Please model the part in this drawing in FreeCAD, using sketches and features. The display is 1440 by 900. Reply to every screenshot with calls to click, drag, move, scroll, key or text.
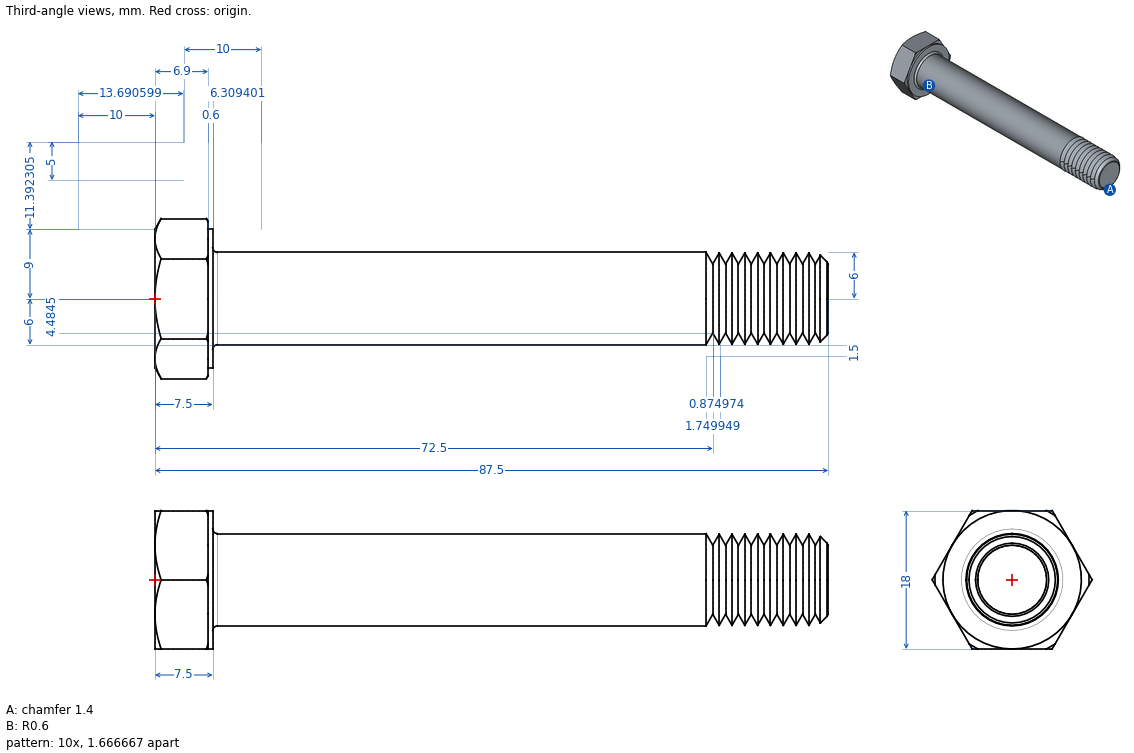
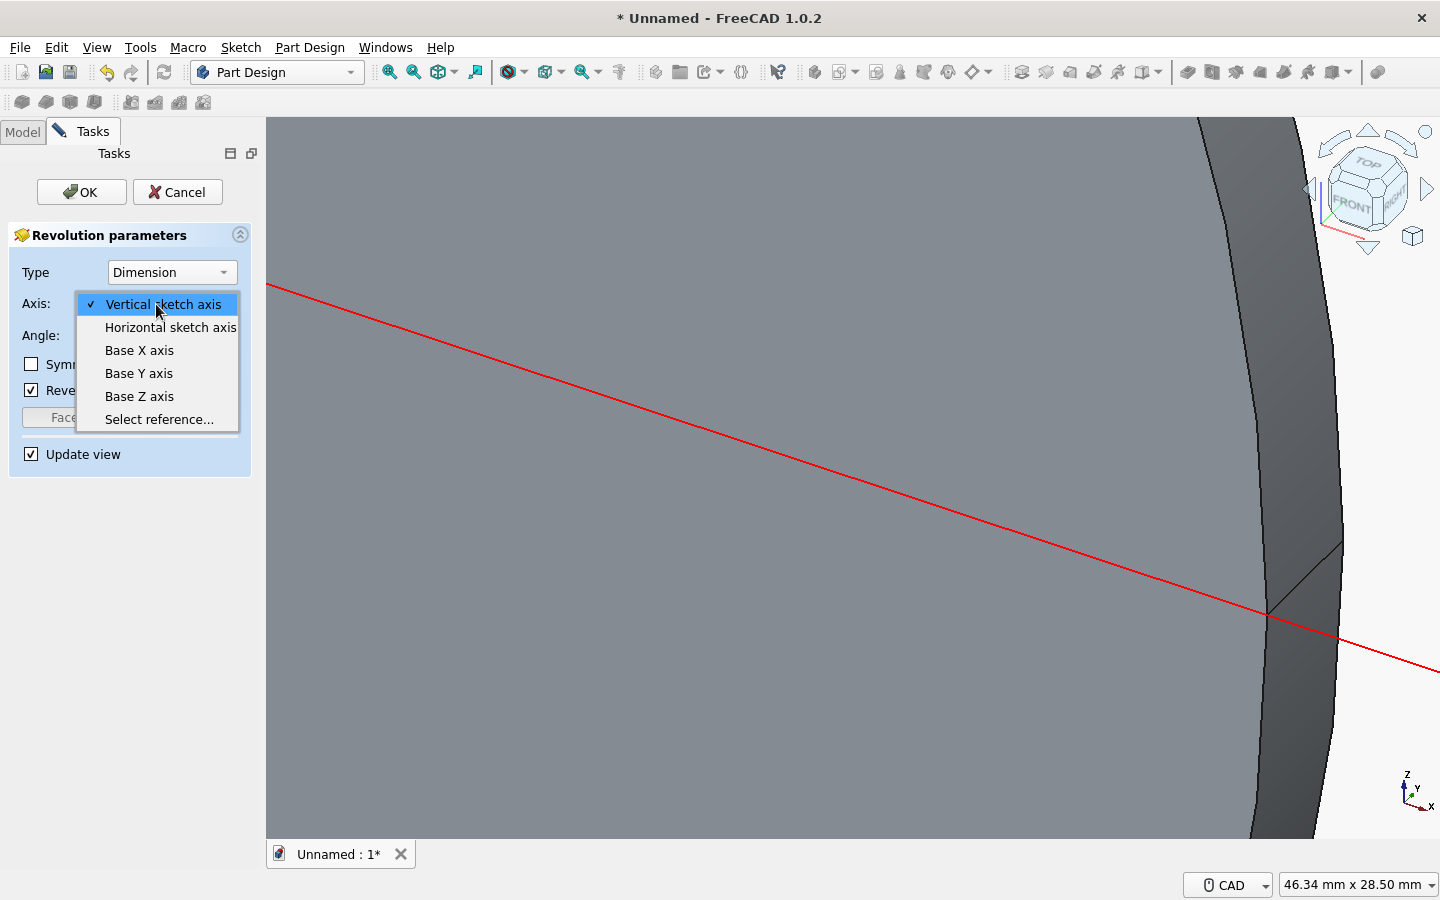
click(156, 328)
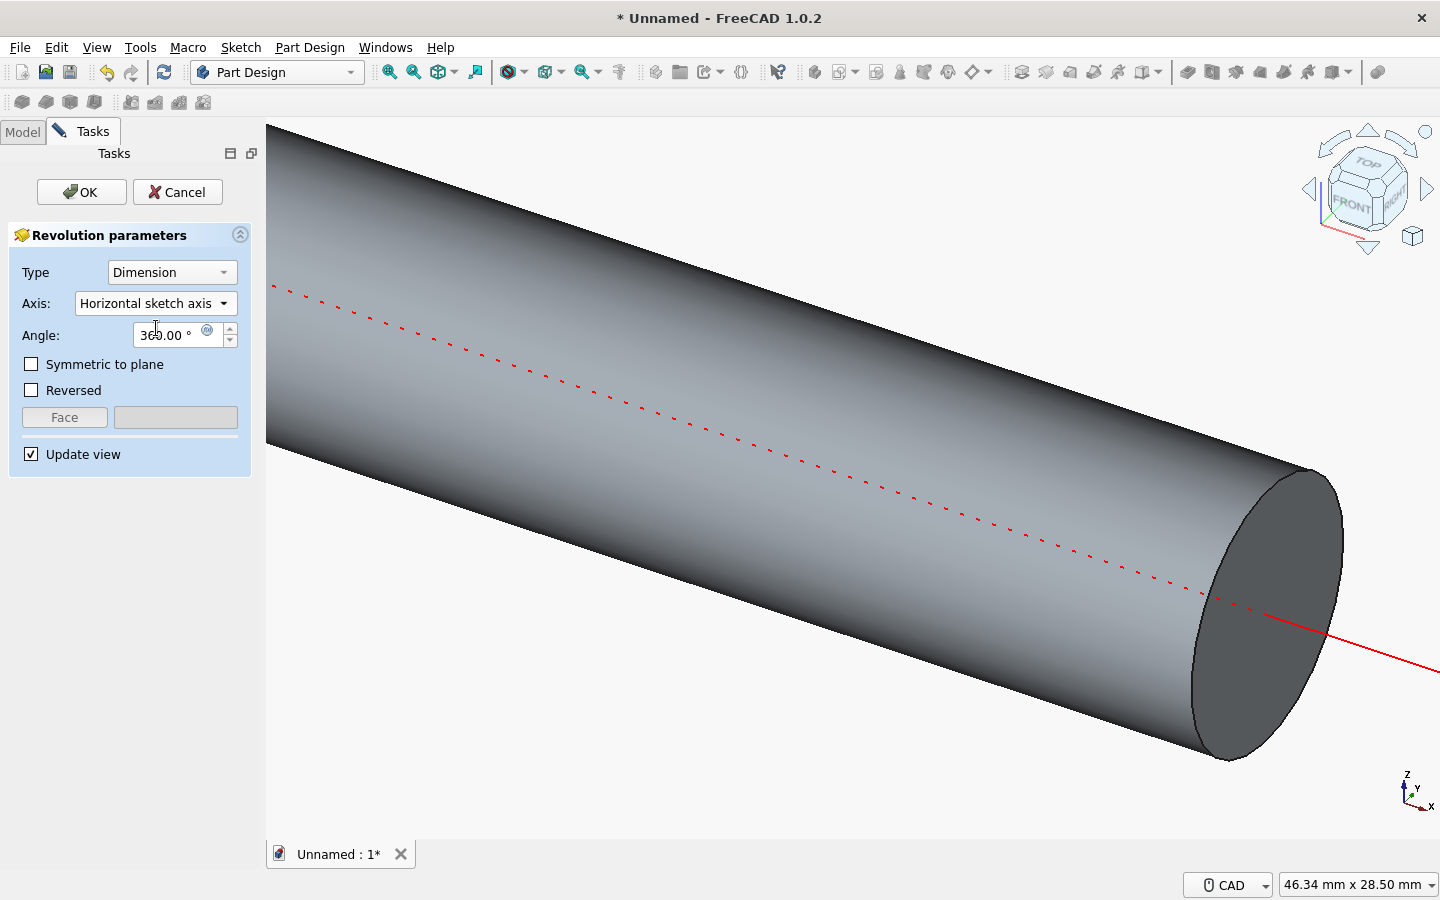
click(82, 192)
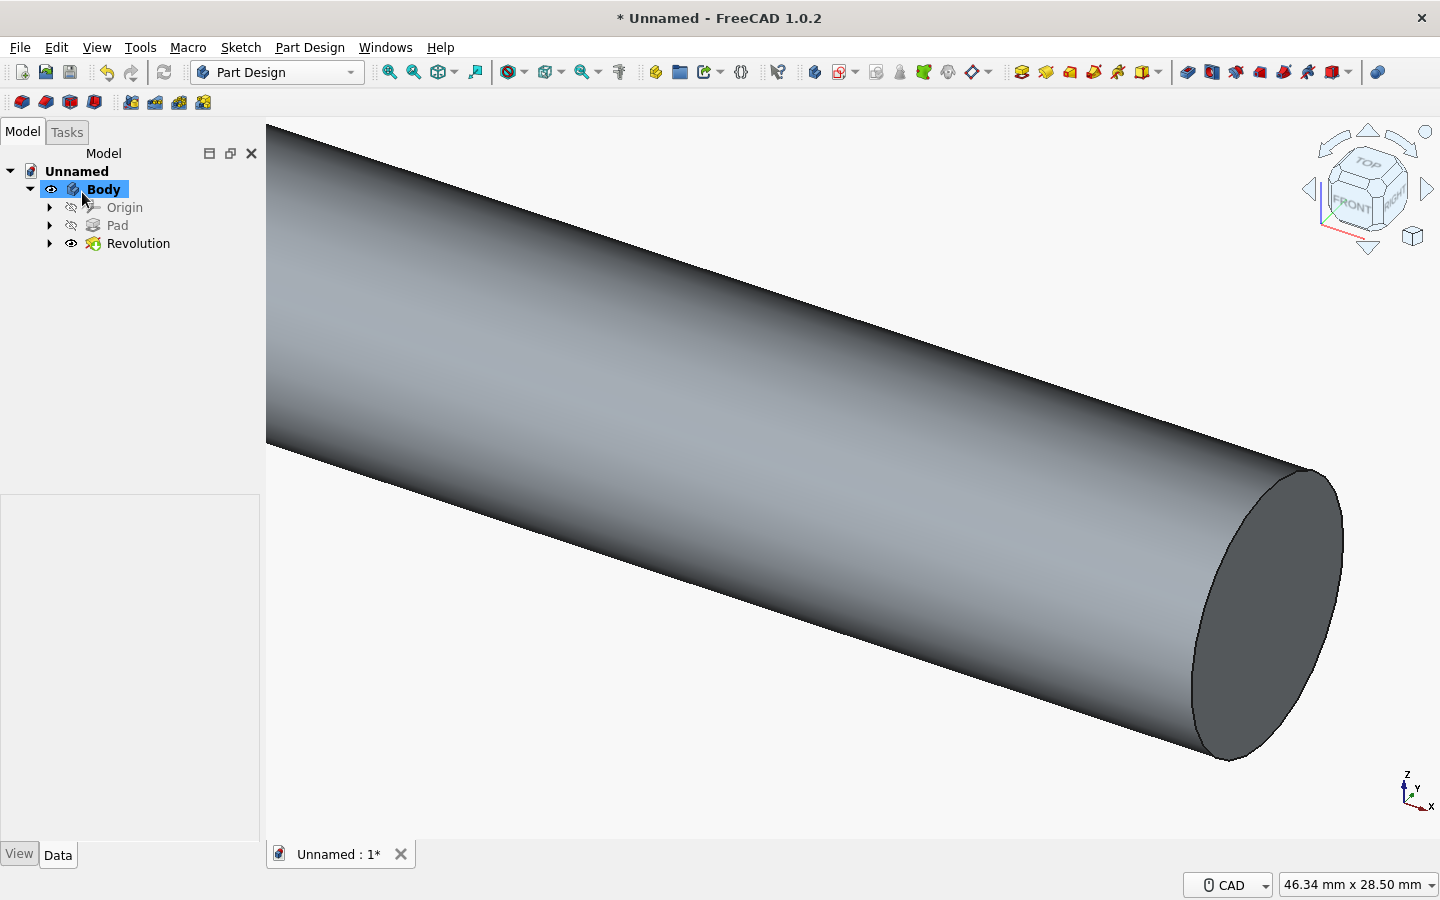
click(390, 72)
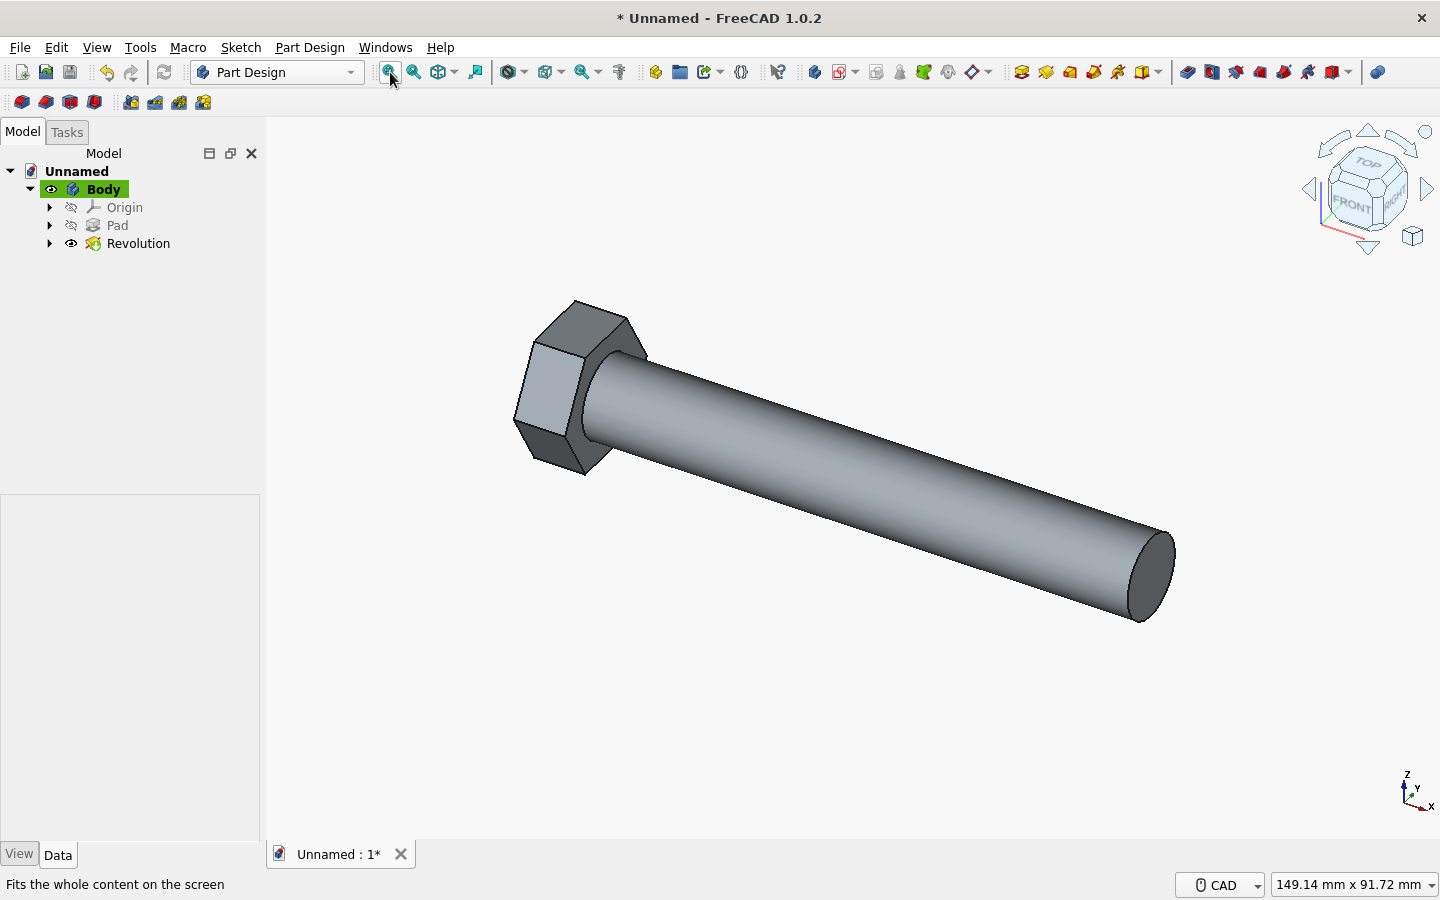
click(840, 72)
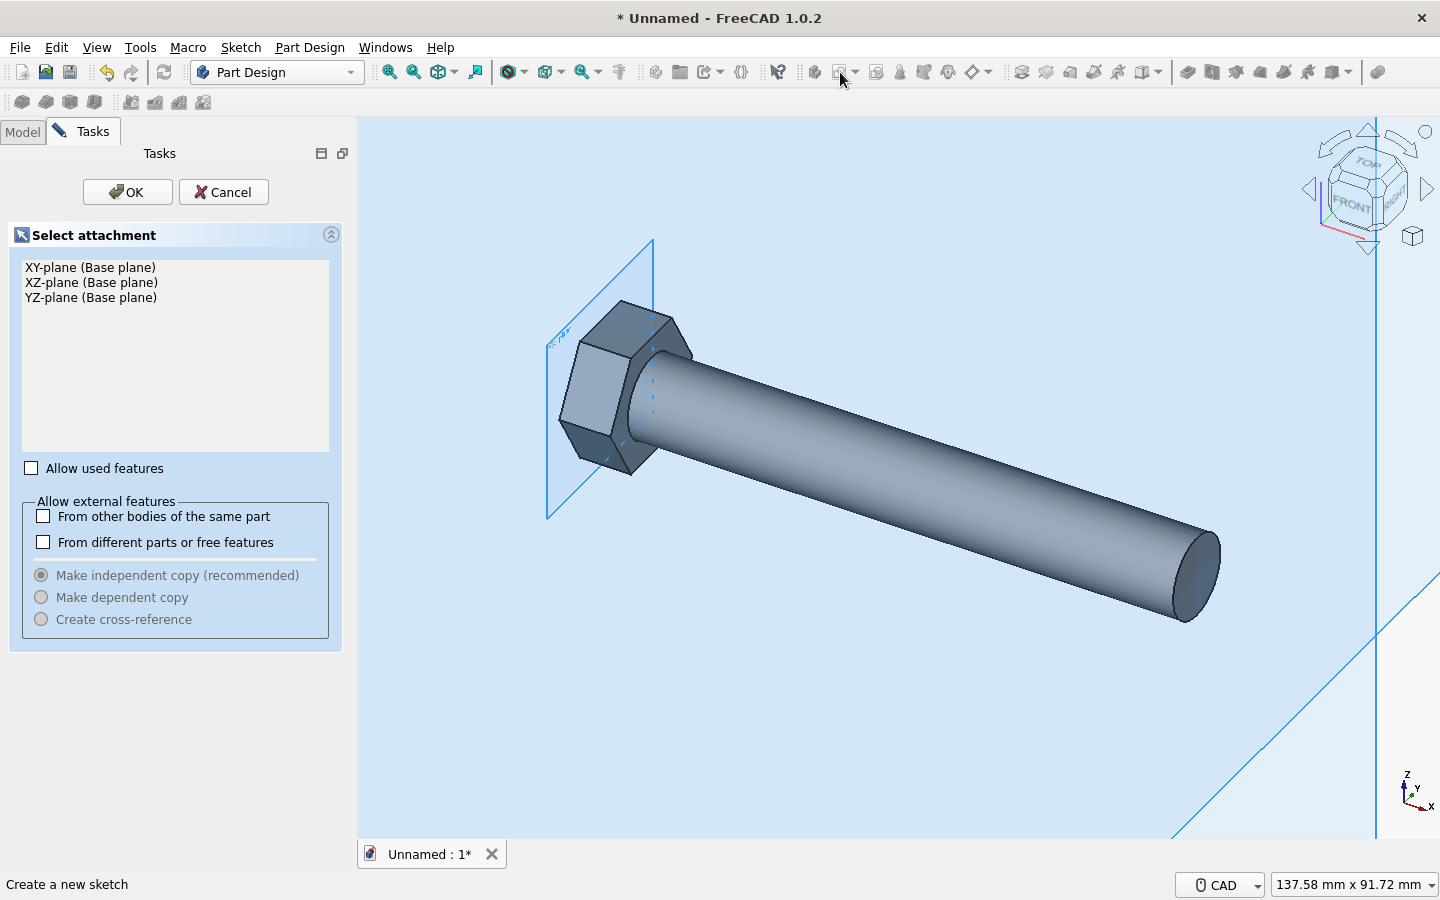
click(82, 268)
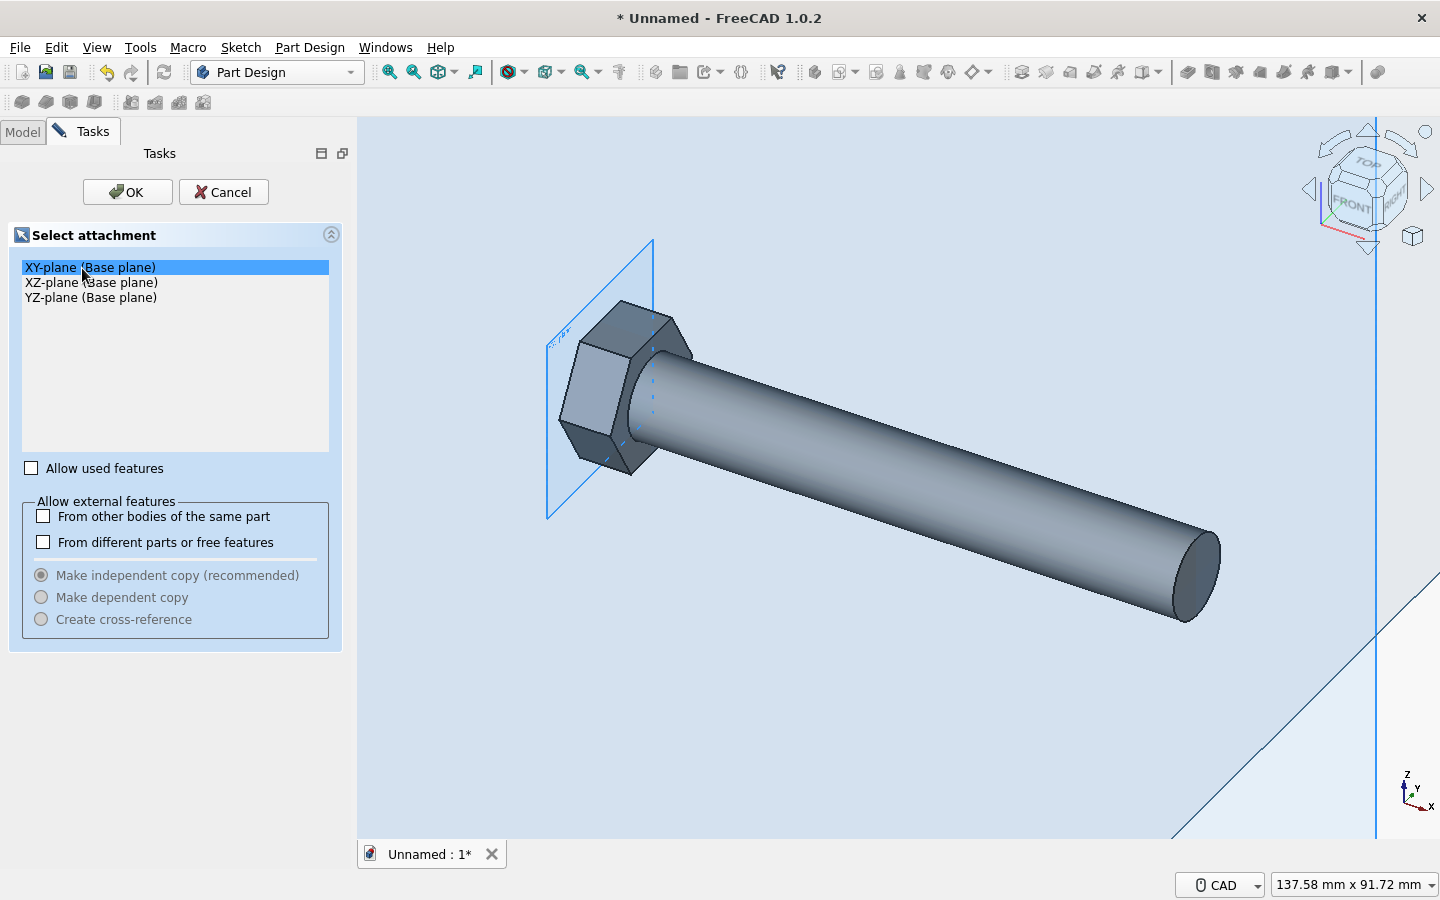
click(128, 192)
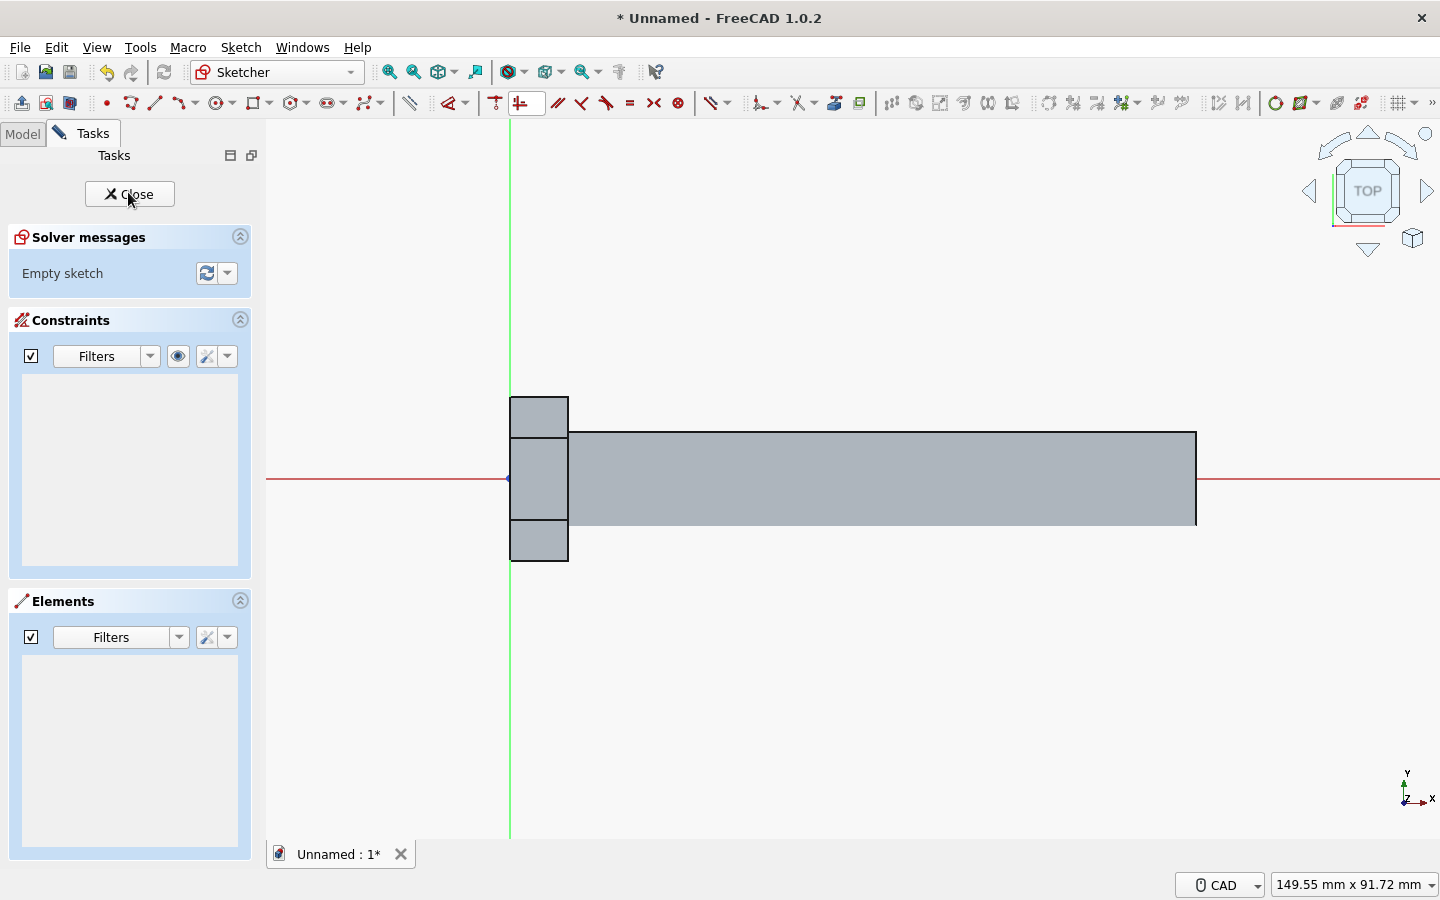
click(70, 104)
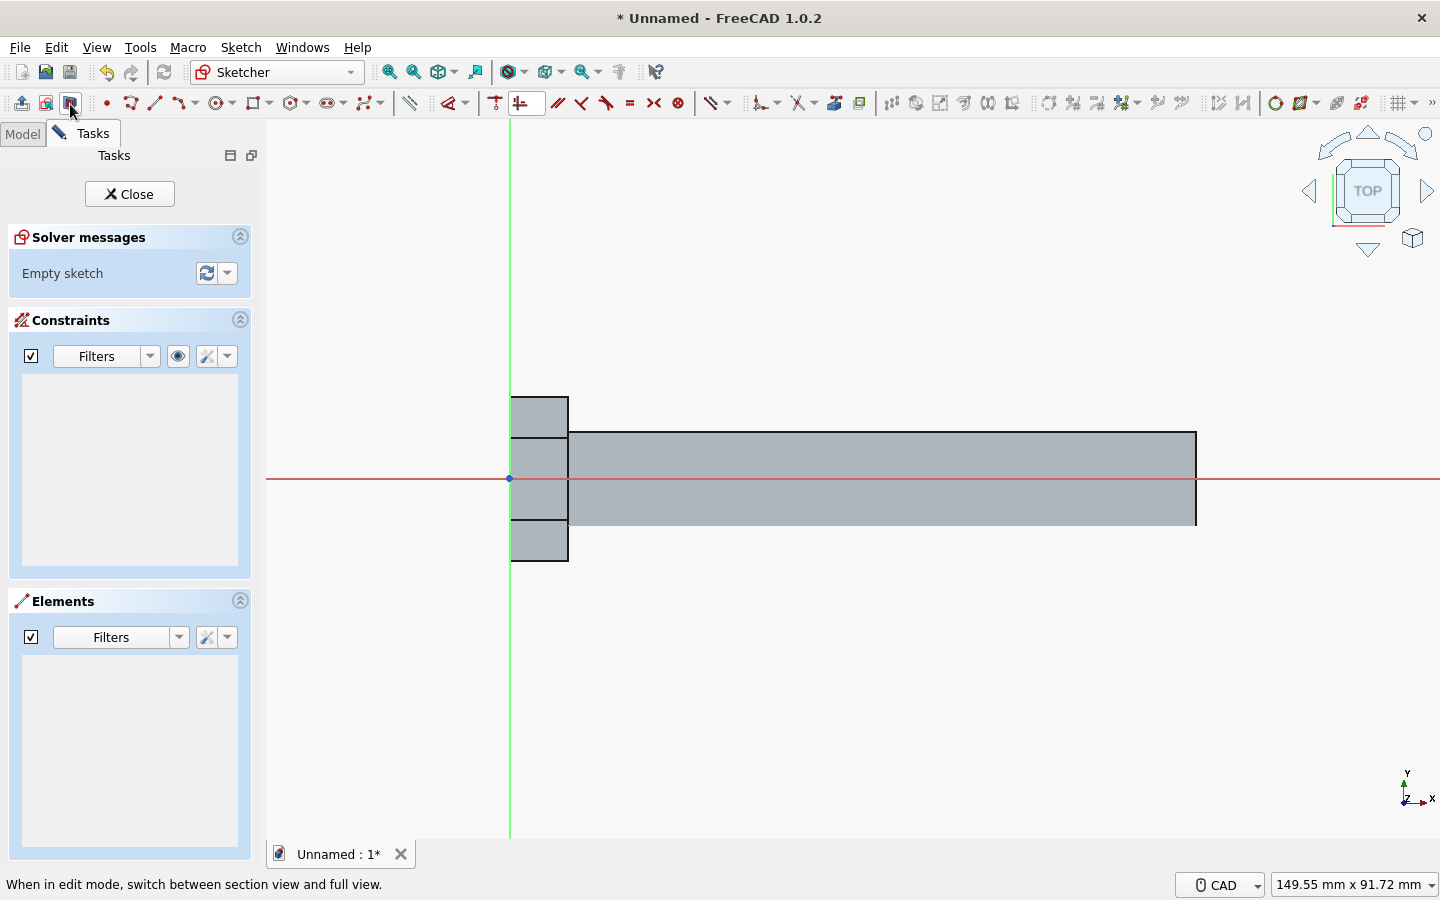
scroll(310, 352, up, 5)